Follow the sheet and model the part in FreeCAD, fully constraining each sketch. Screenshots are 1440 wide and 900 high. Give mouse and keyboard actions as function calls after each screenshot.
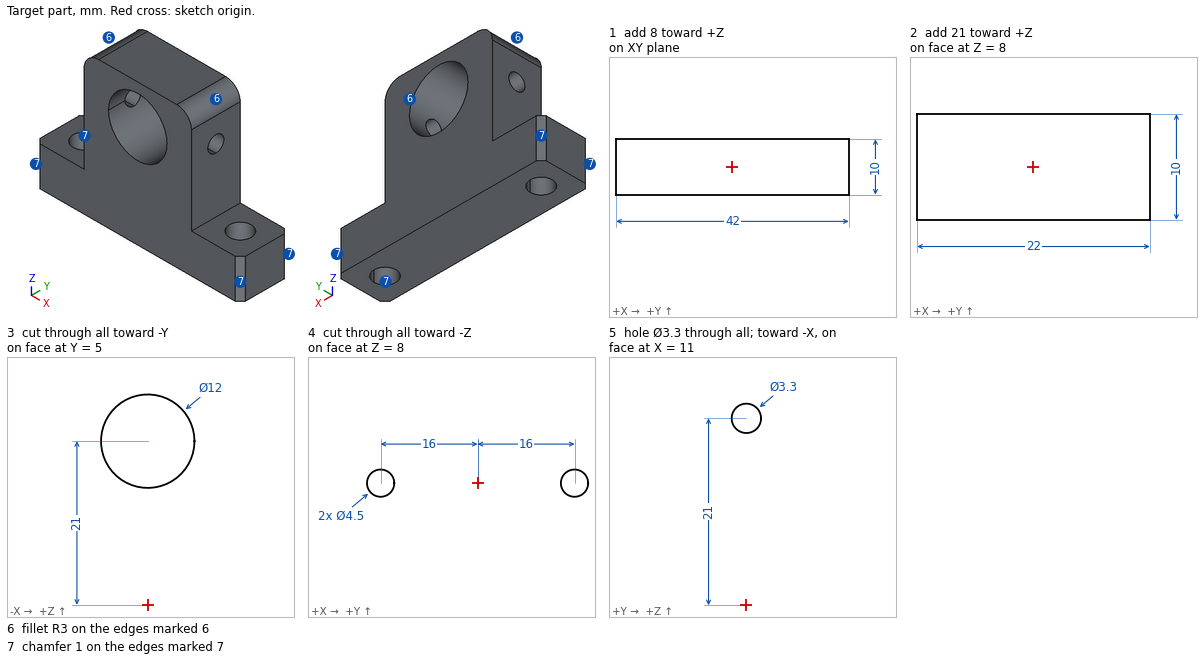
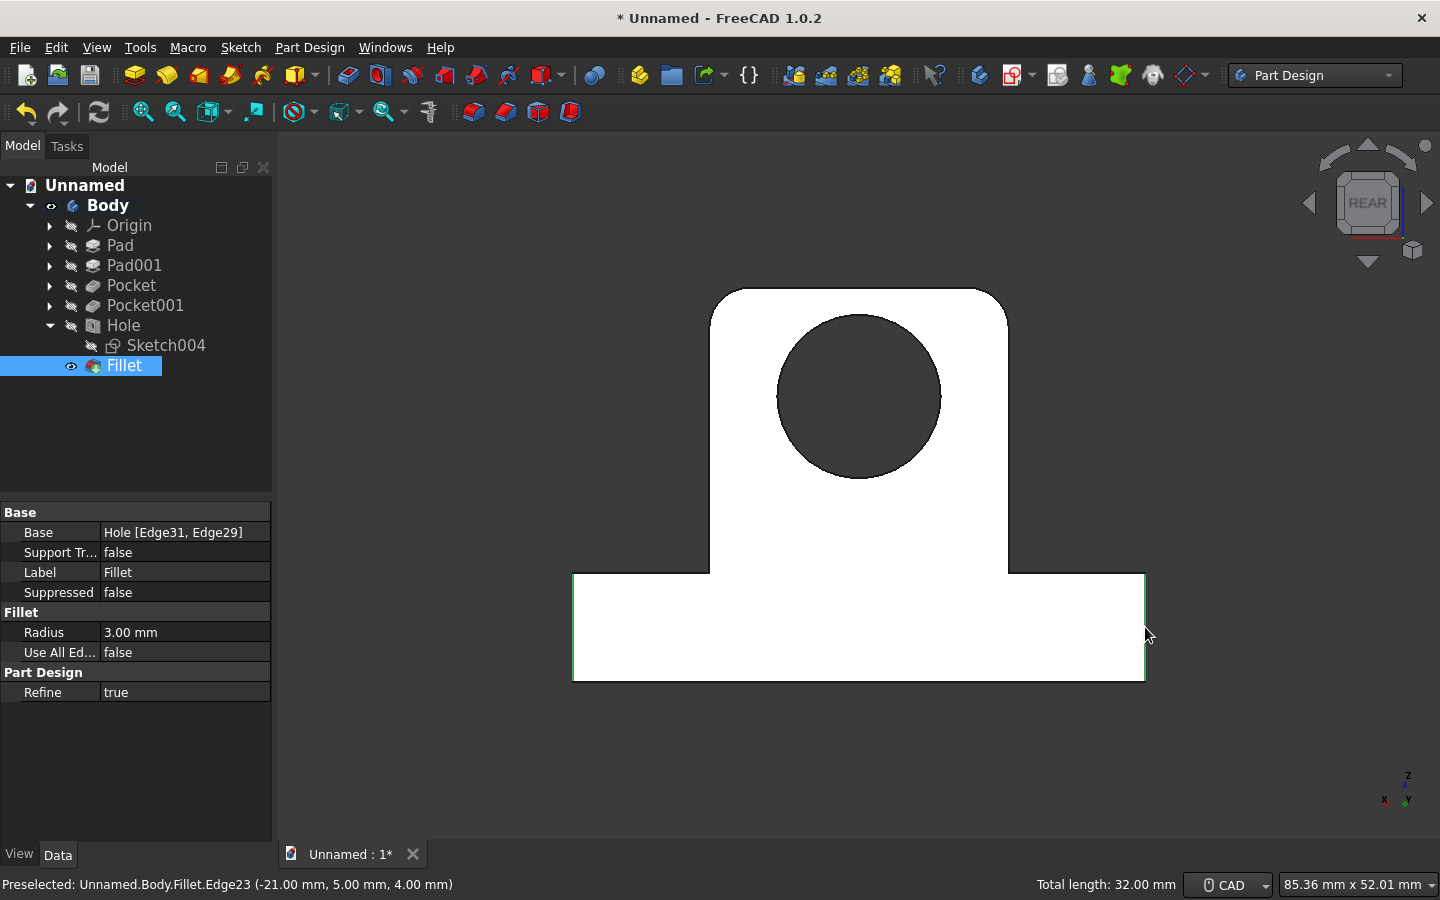
click(506, 112)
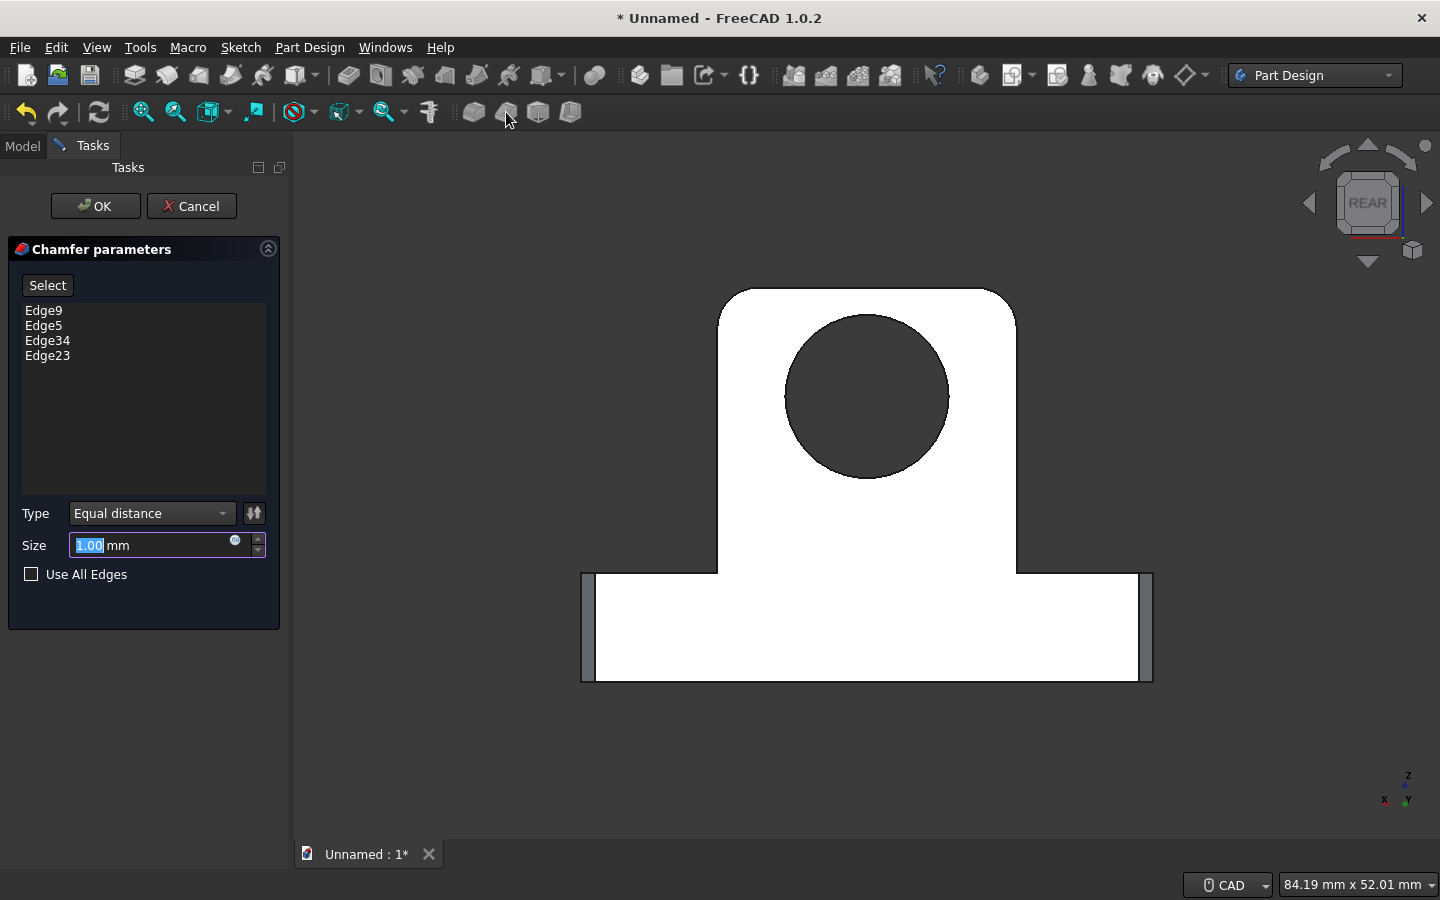
text(1)
key(Tab)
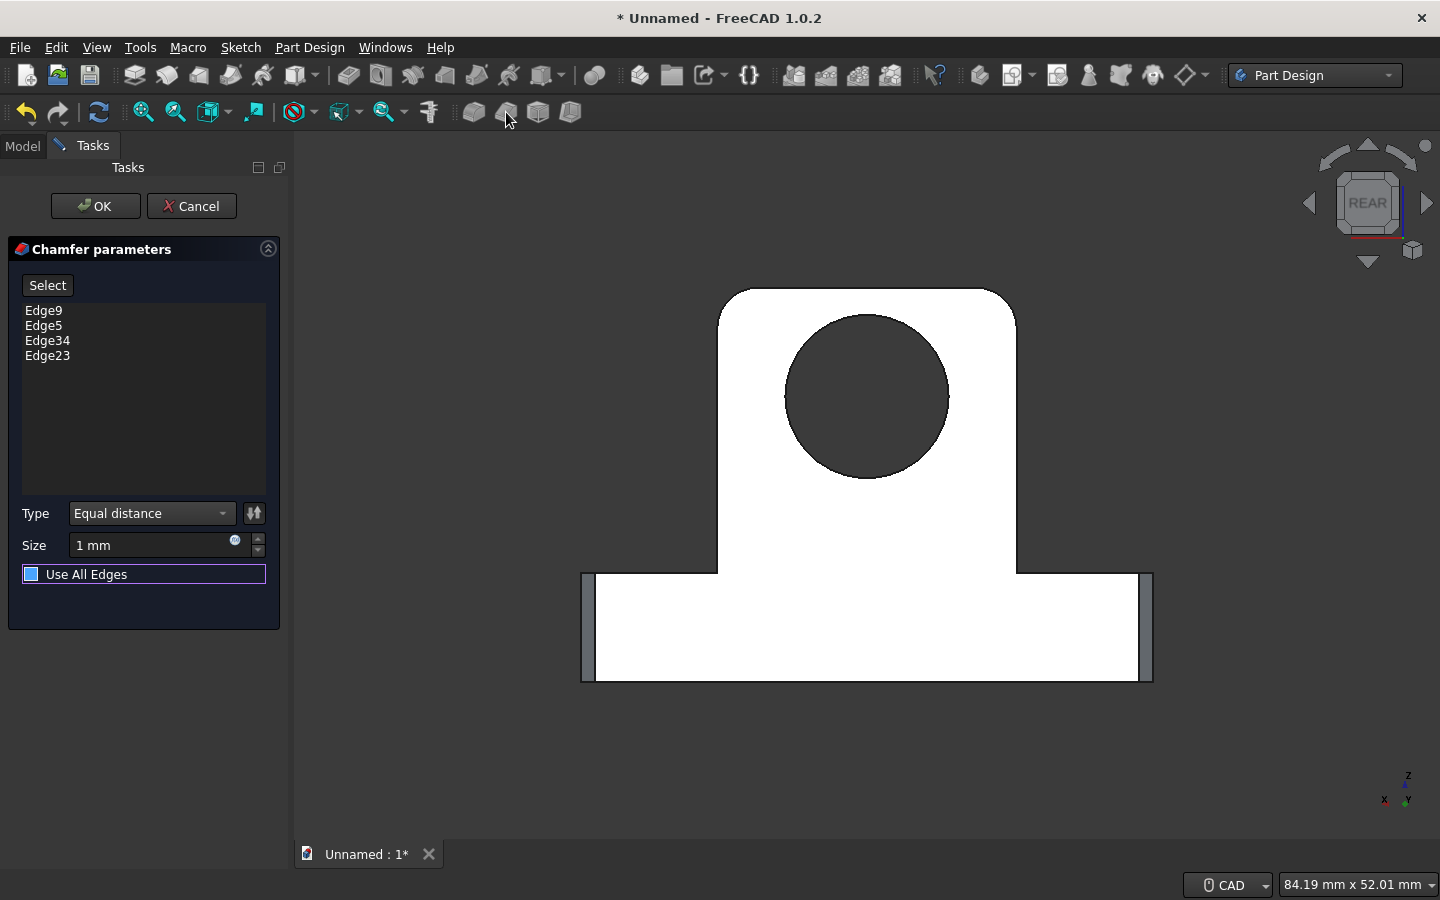
click(96, 206)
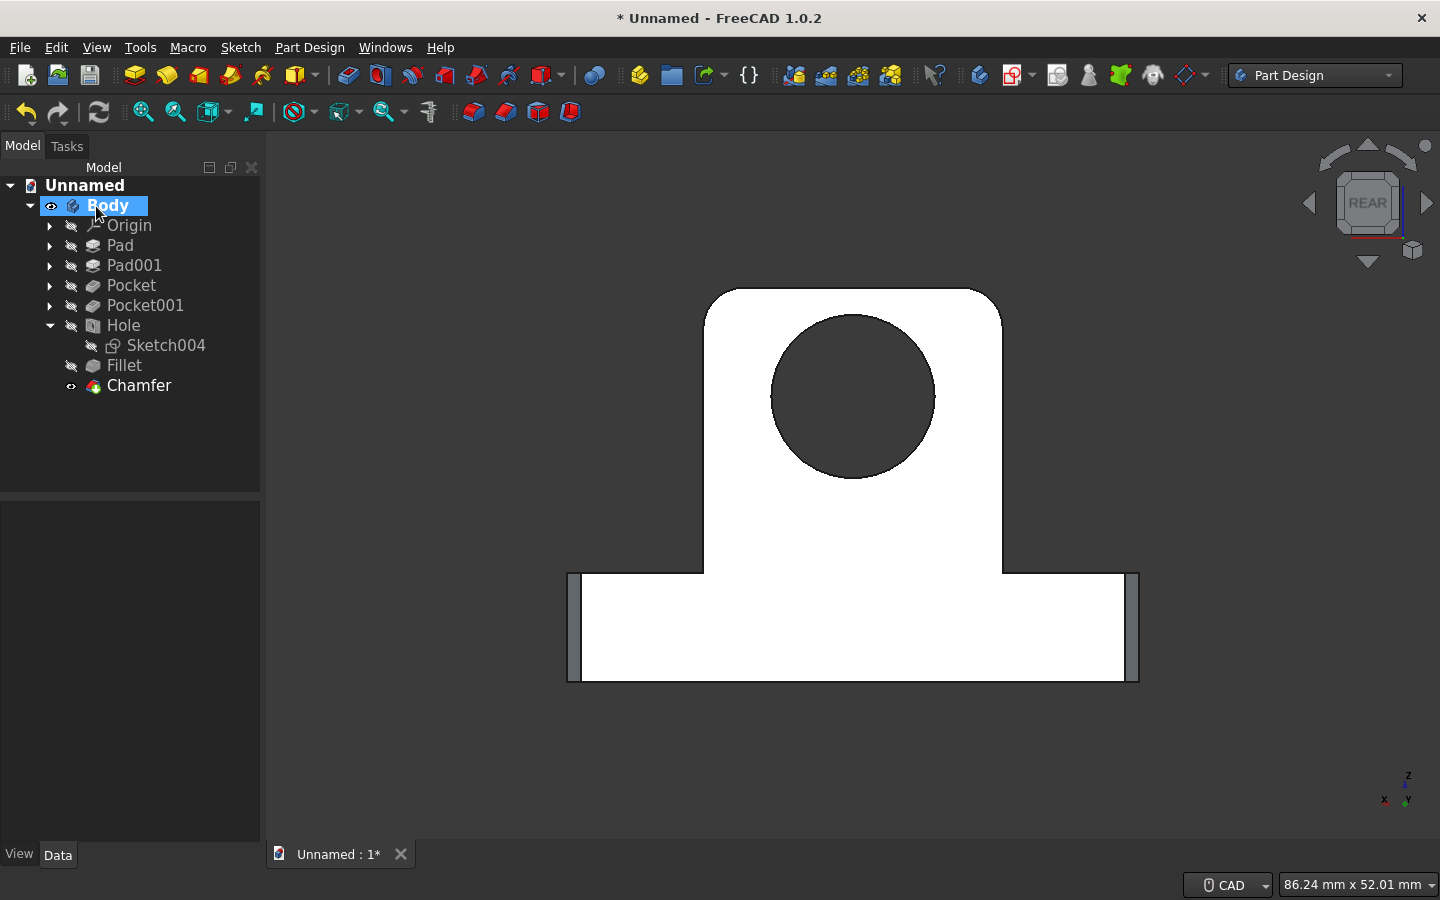
key(0)